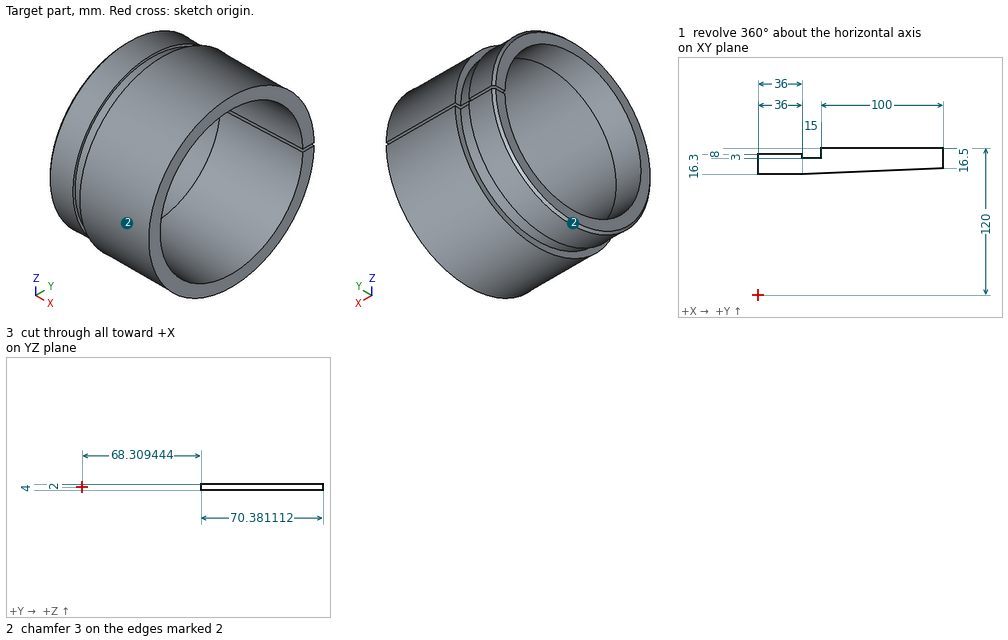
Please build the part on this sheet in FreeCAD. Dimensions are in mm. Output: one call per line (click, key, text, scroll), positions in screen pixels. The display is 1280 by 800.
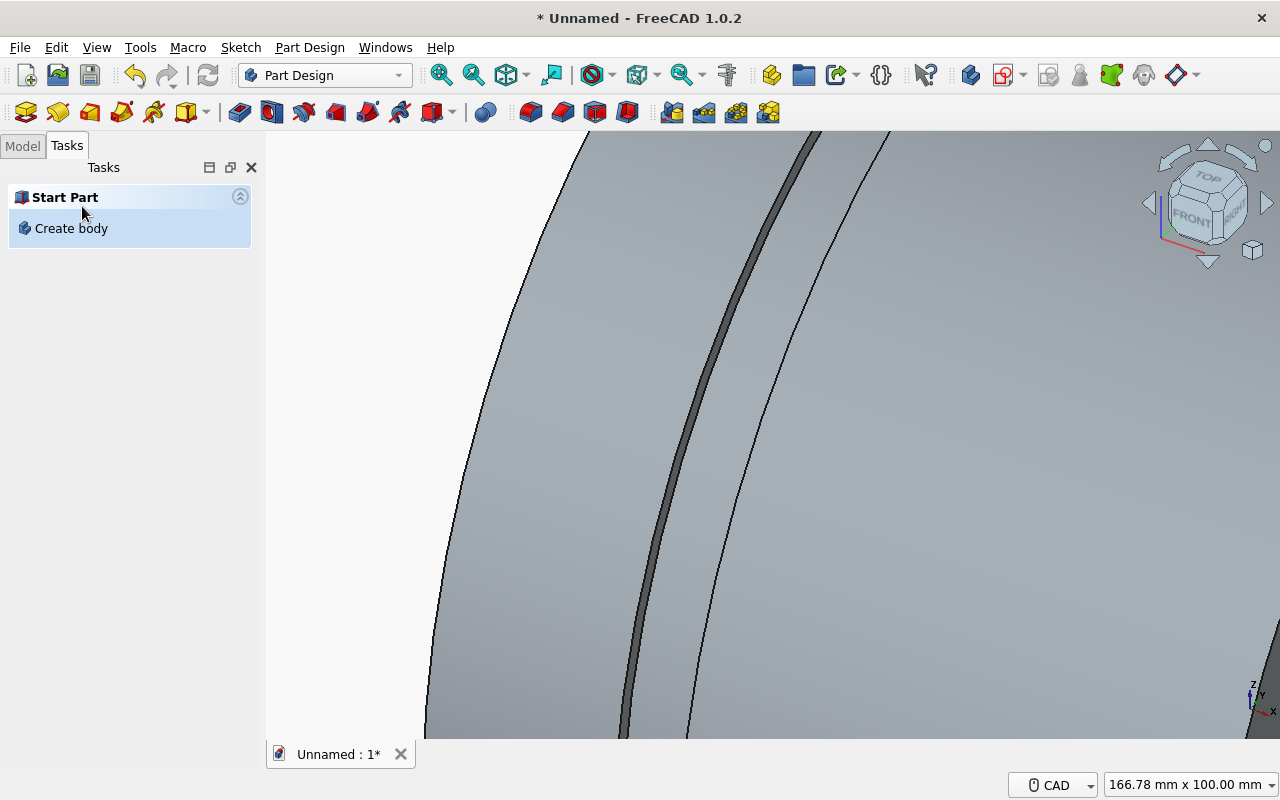
click(442, 76)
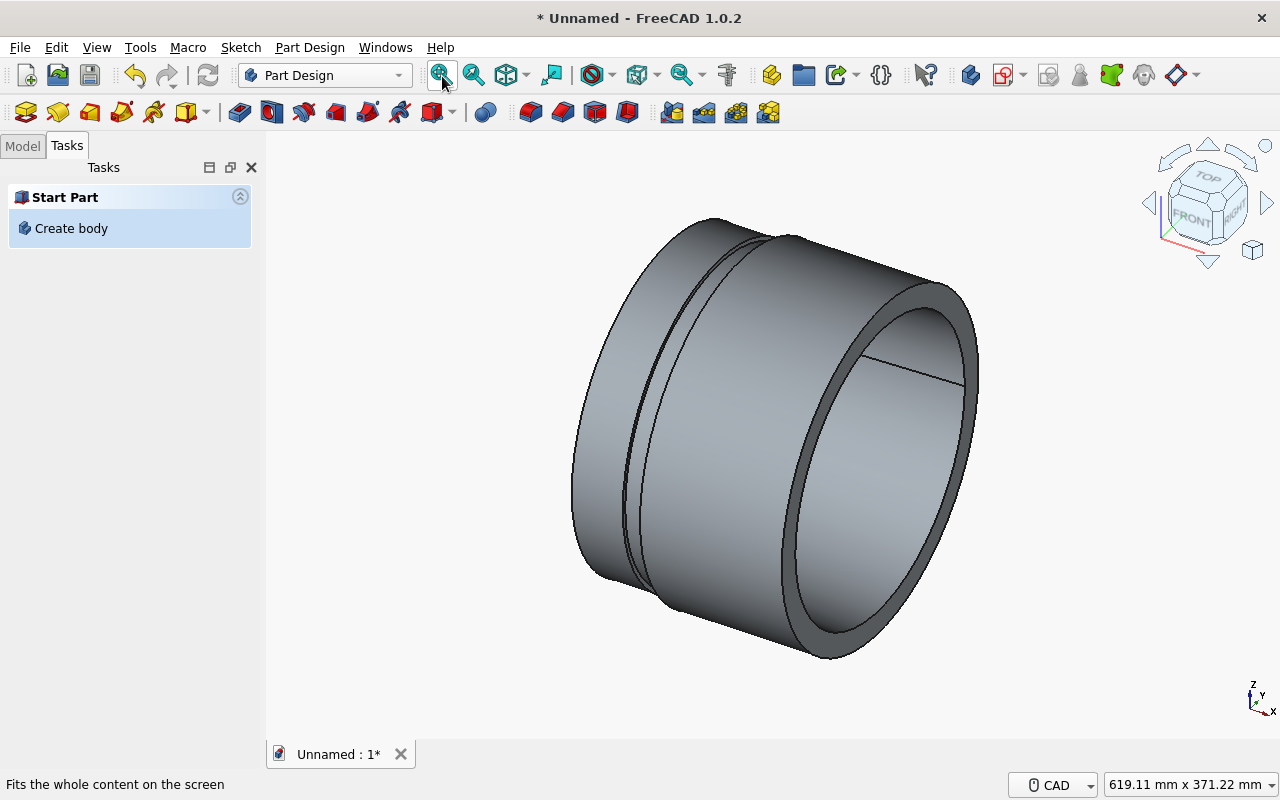
key(0)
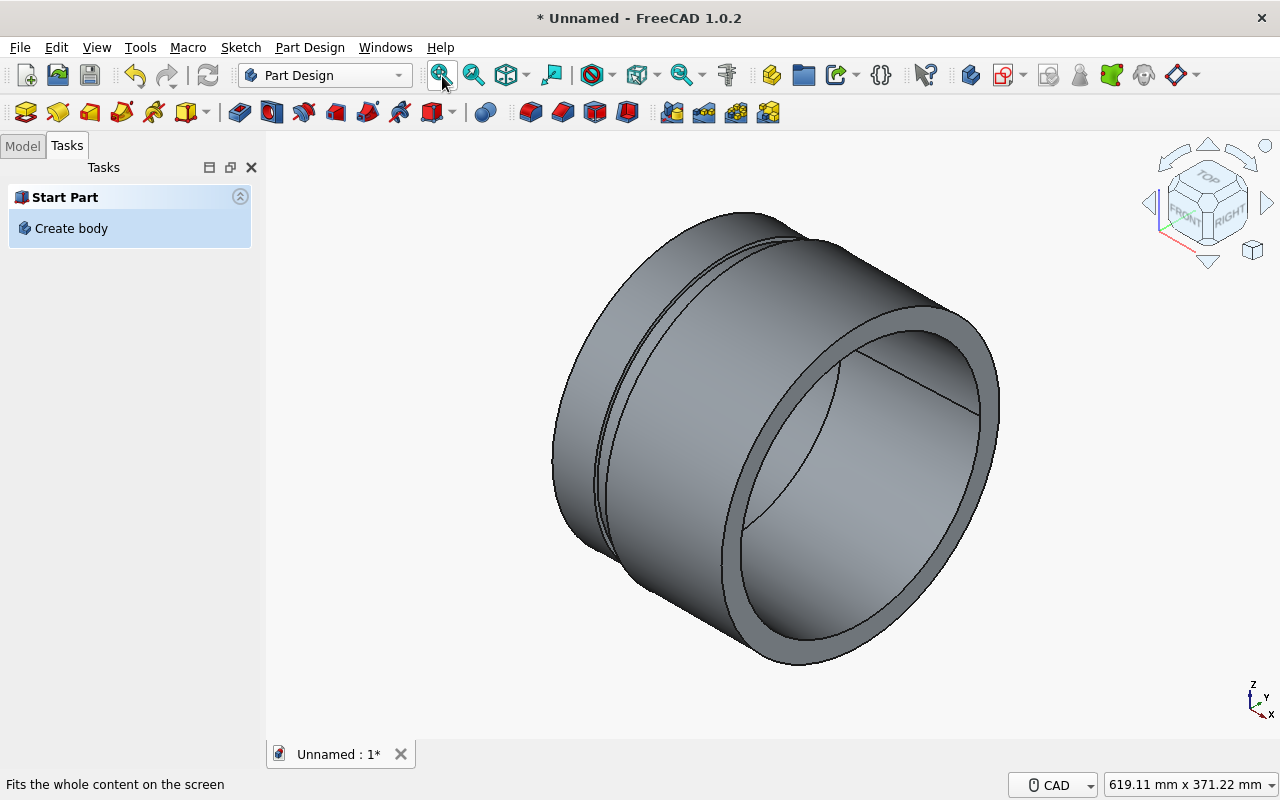
key(2)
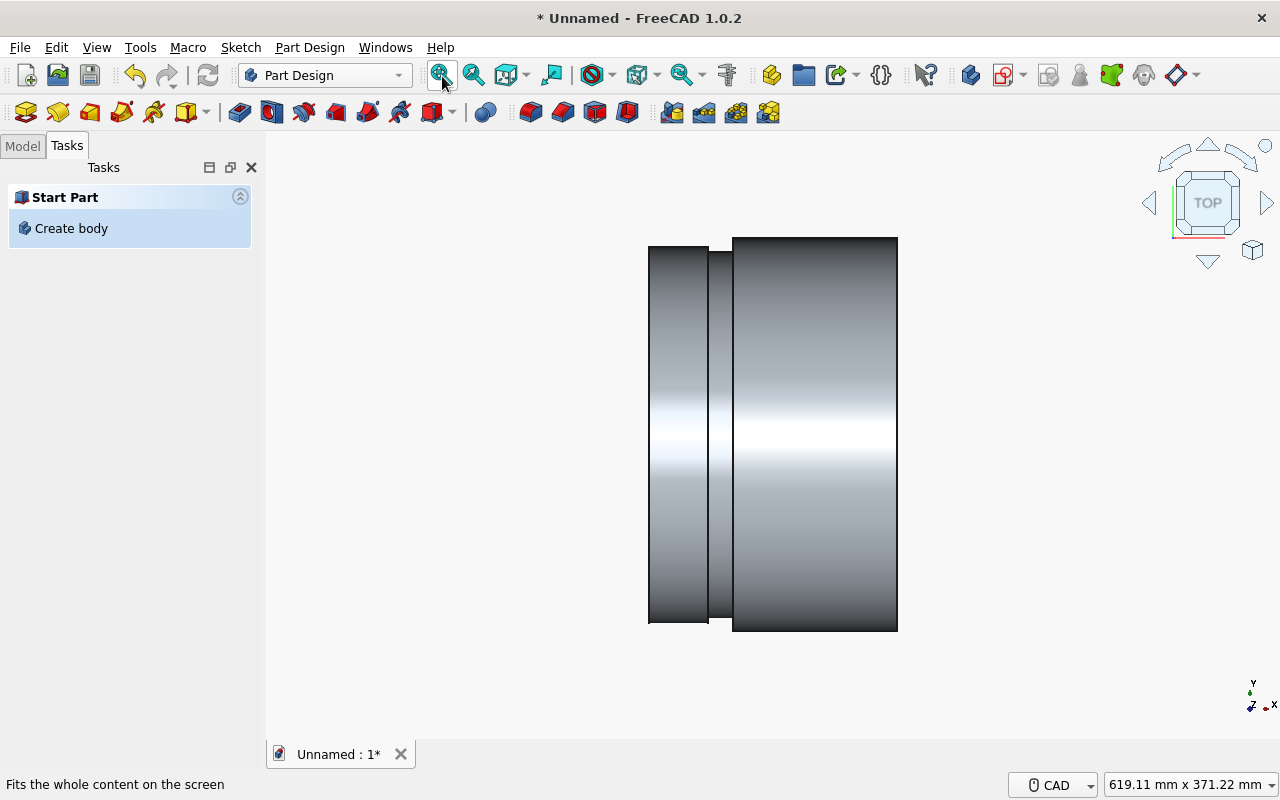
click(649, 586)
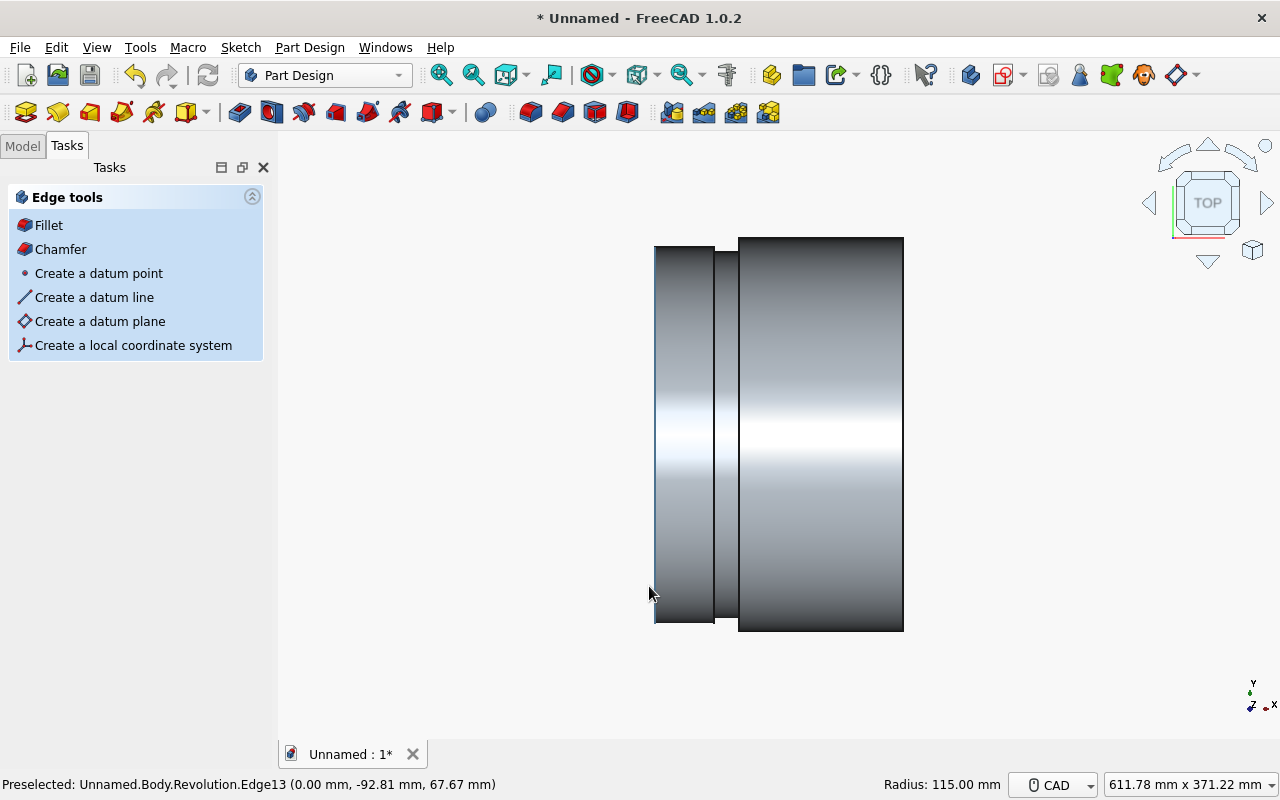
click(564, 112)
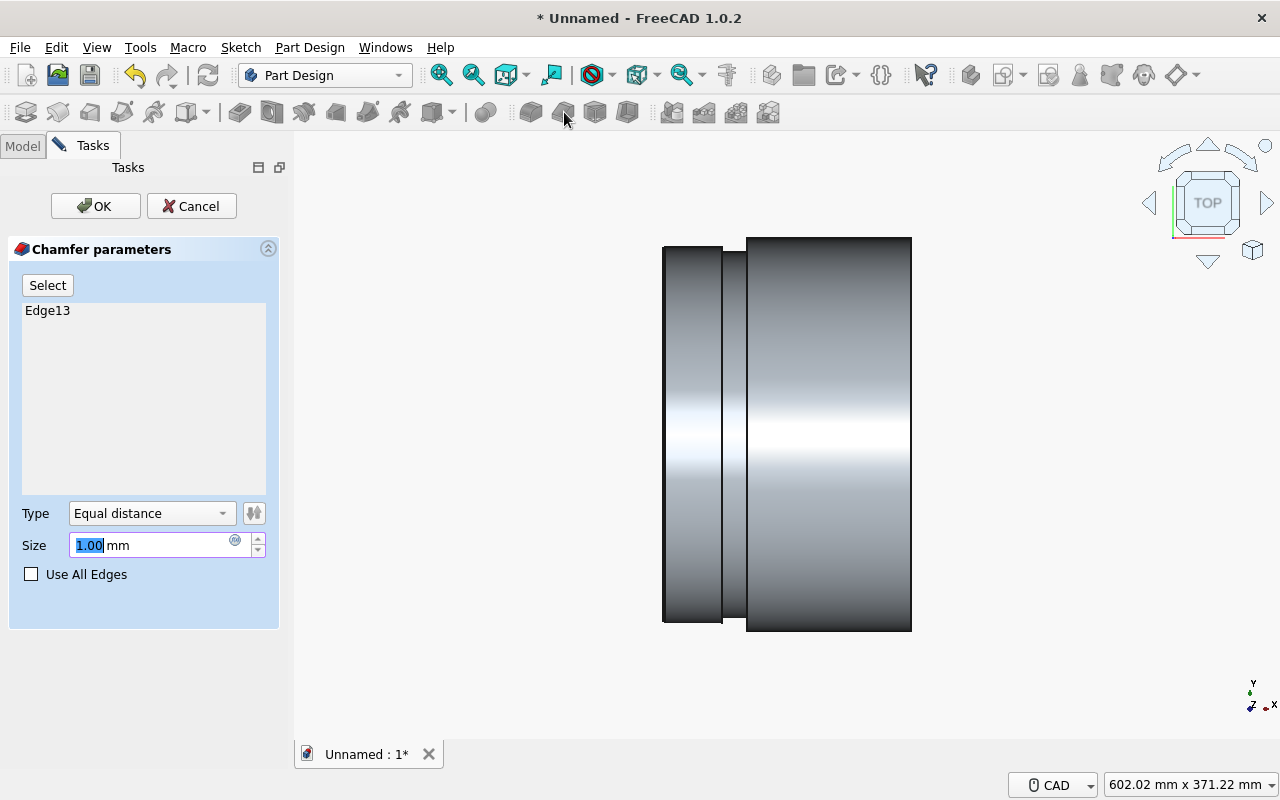
text(3)
key(Tab)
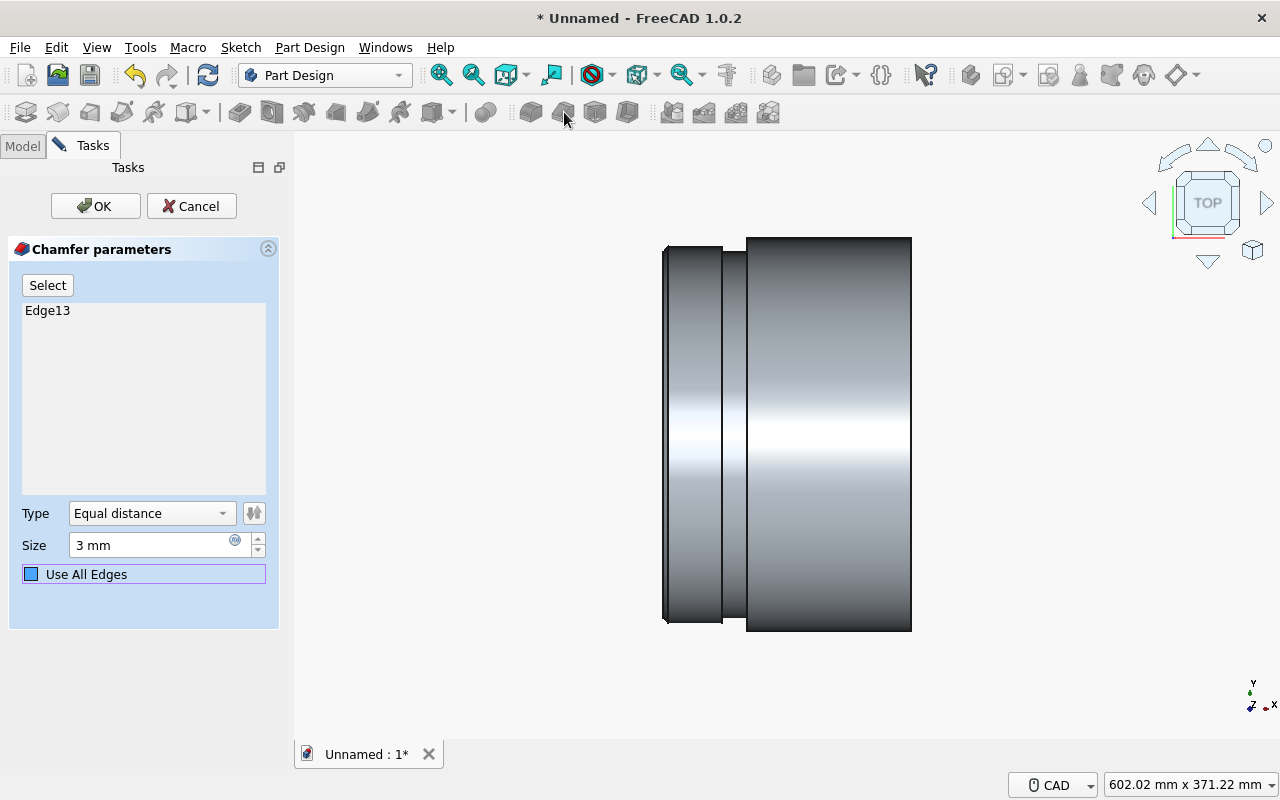
click(96, 206)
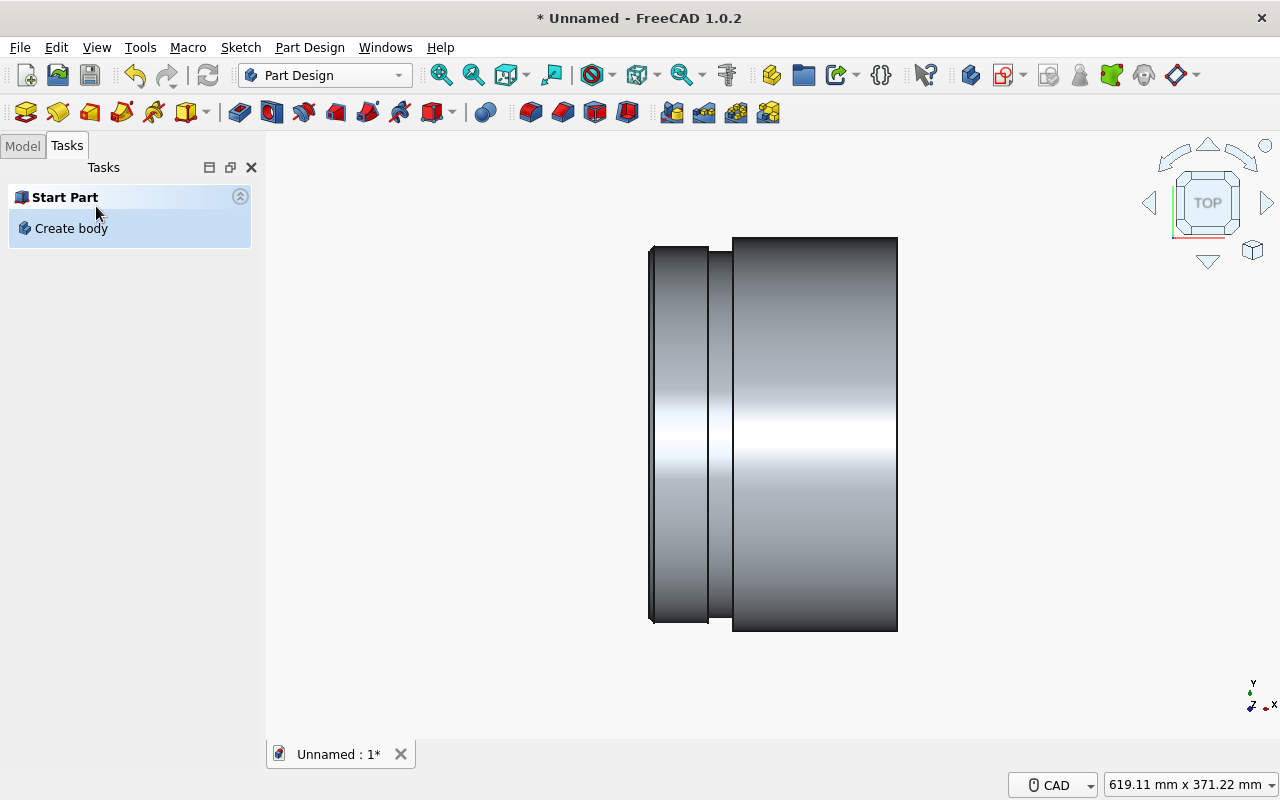
click(1004, 76)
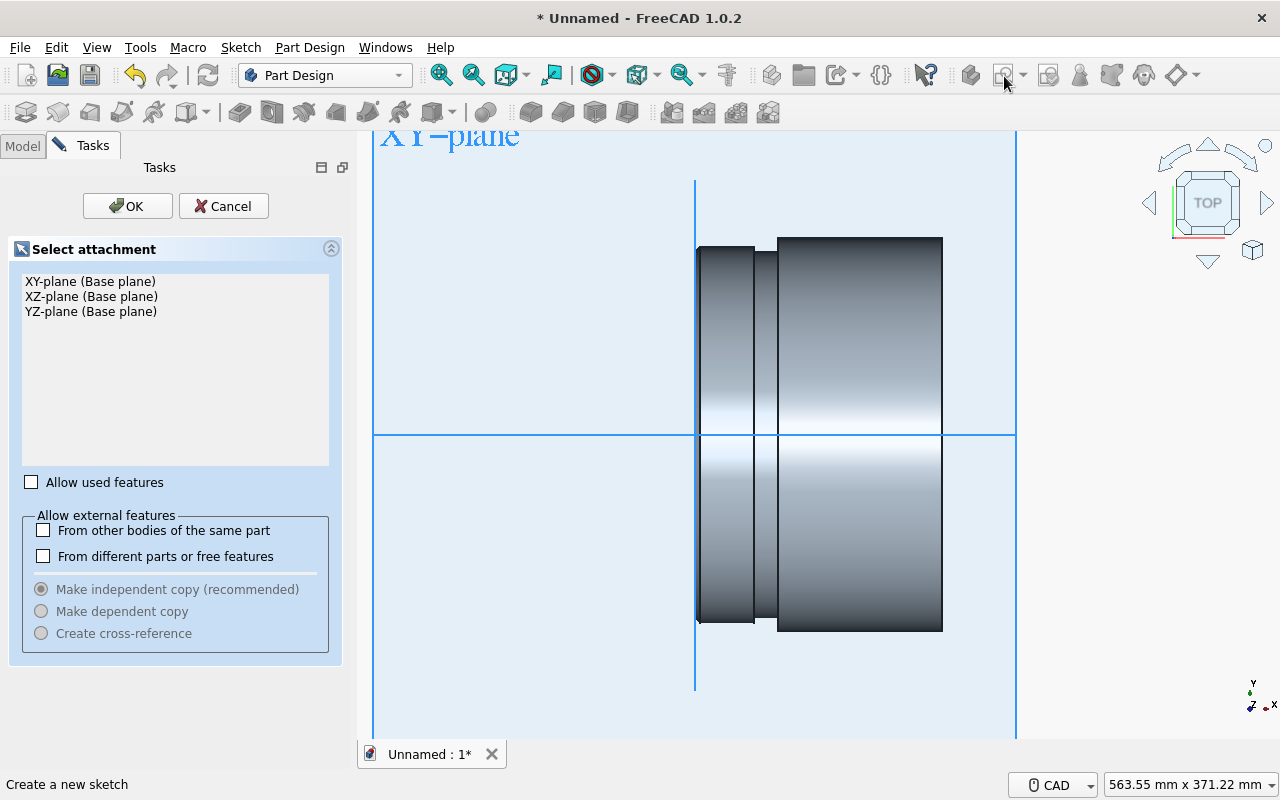
click(82, 312)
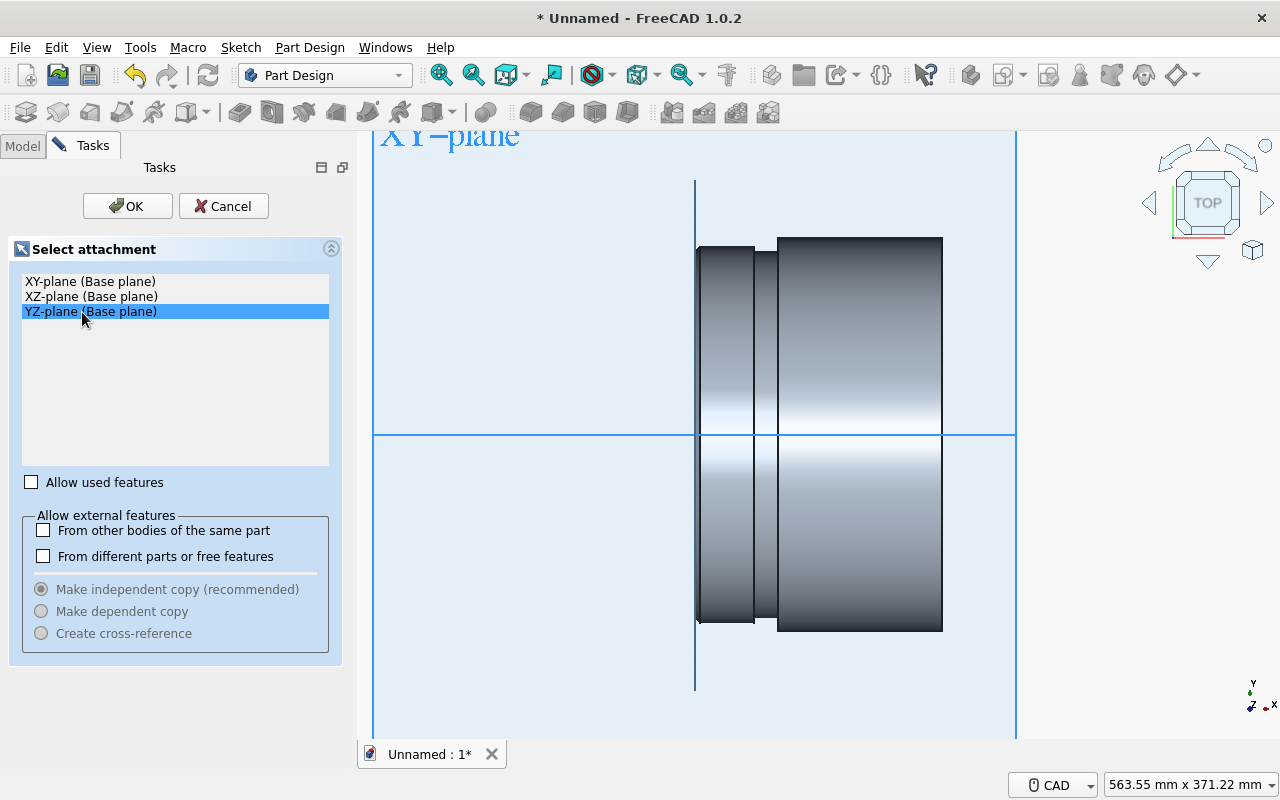
click(128, 206)